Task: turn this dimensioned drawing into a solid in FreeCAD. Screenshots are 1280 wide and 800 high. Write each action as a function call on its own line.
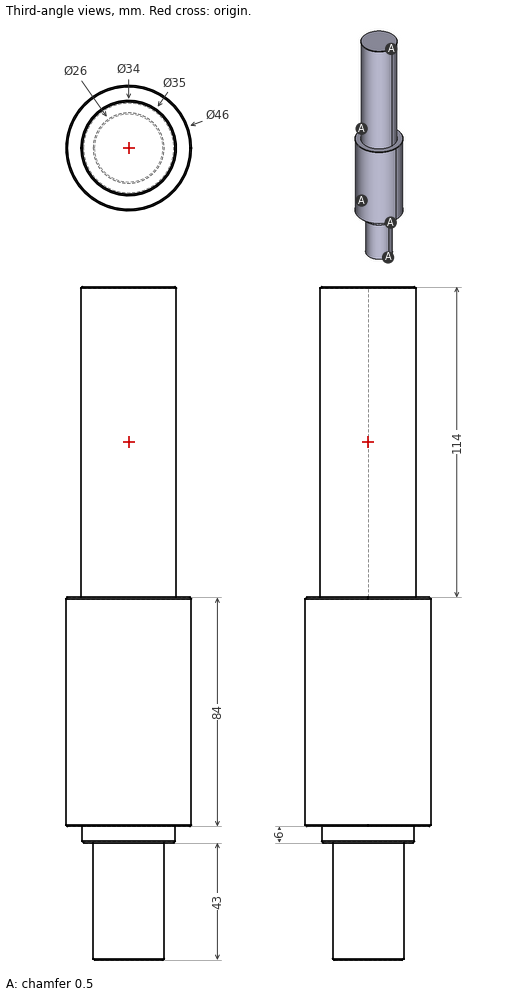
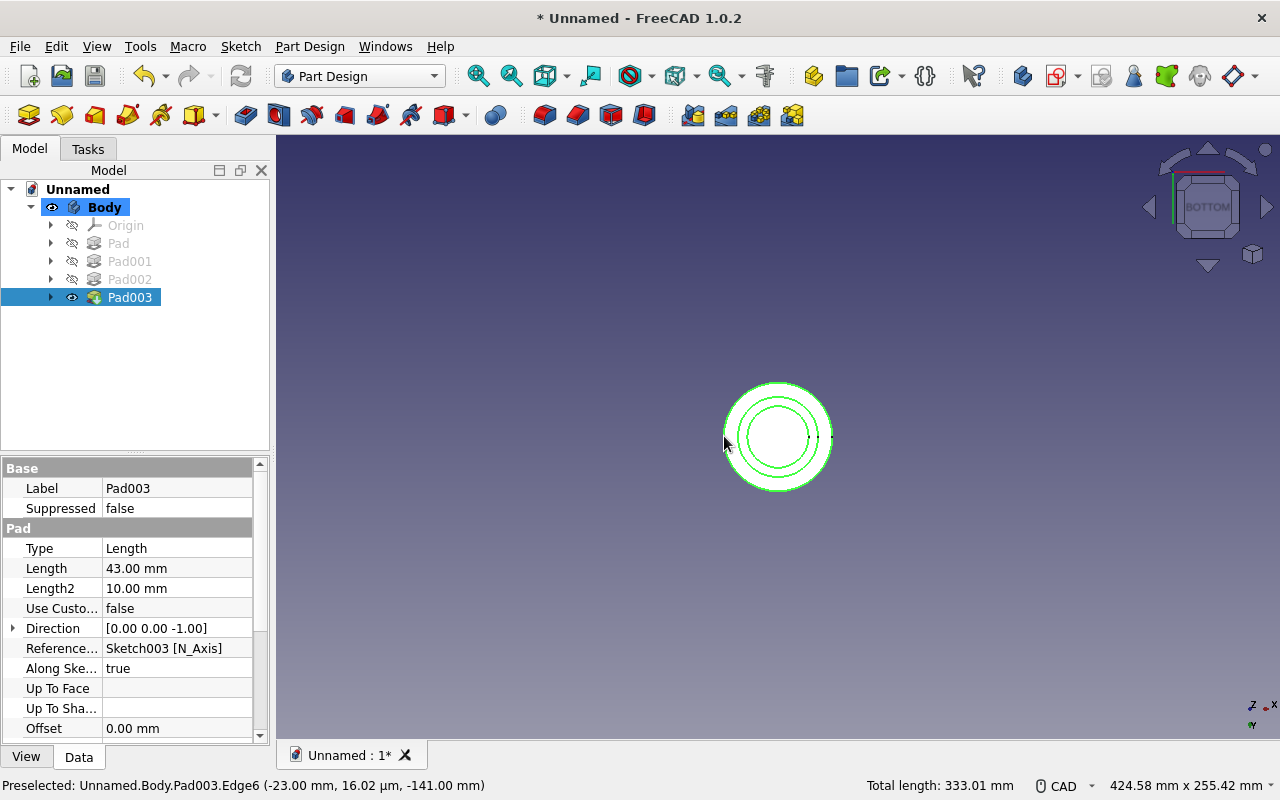
key(0)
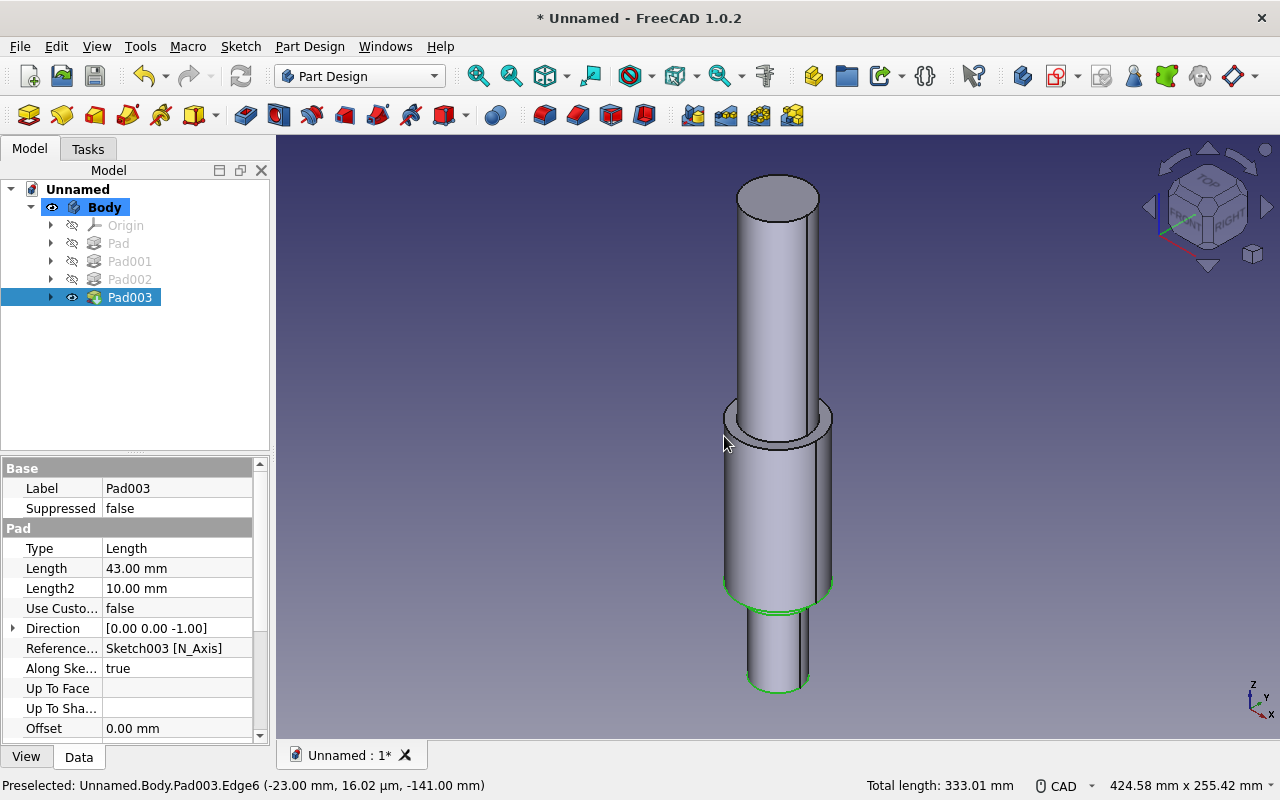
click(797, 176, ctrl)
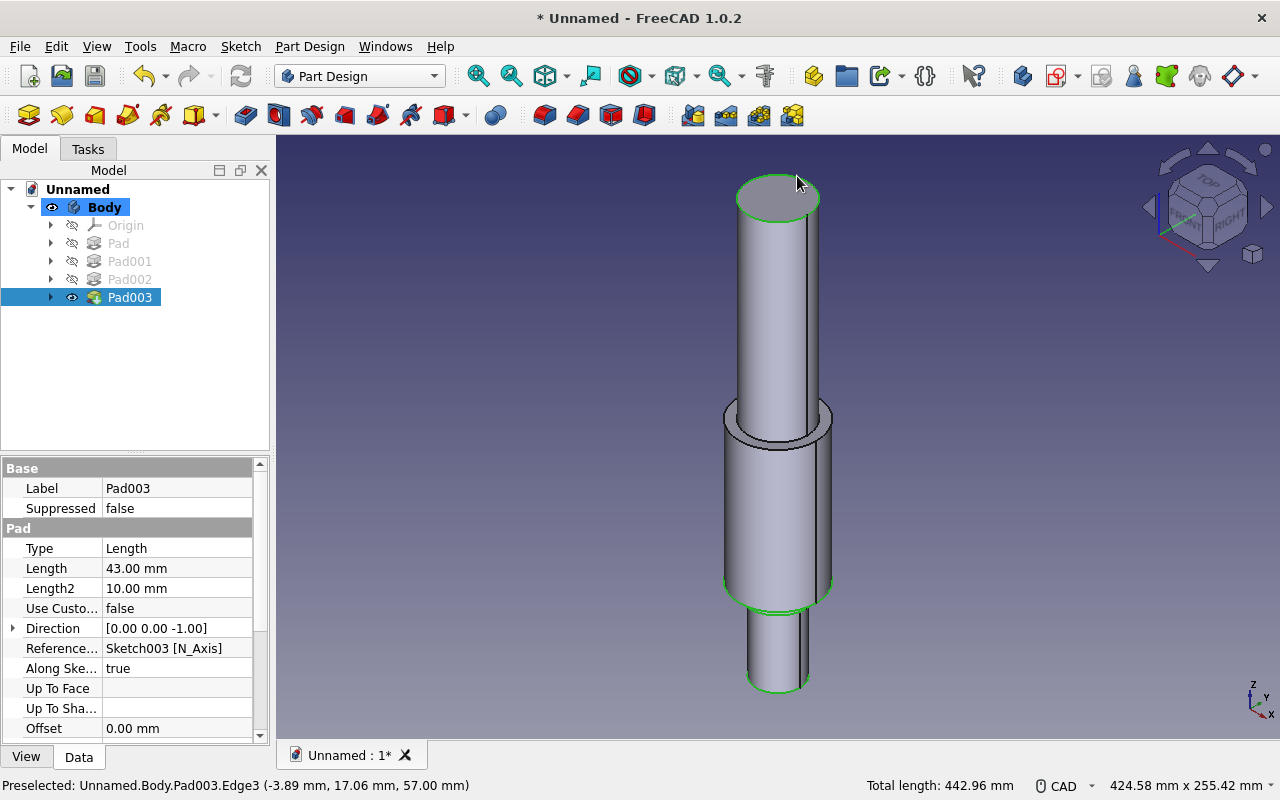
click(730, 432, ctrl)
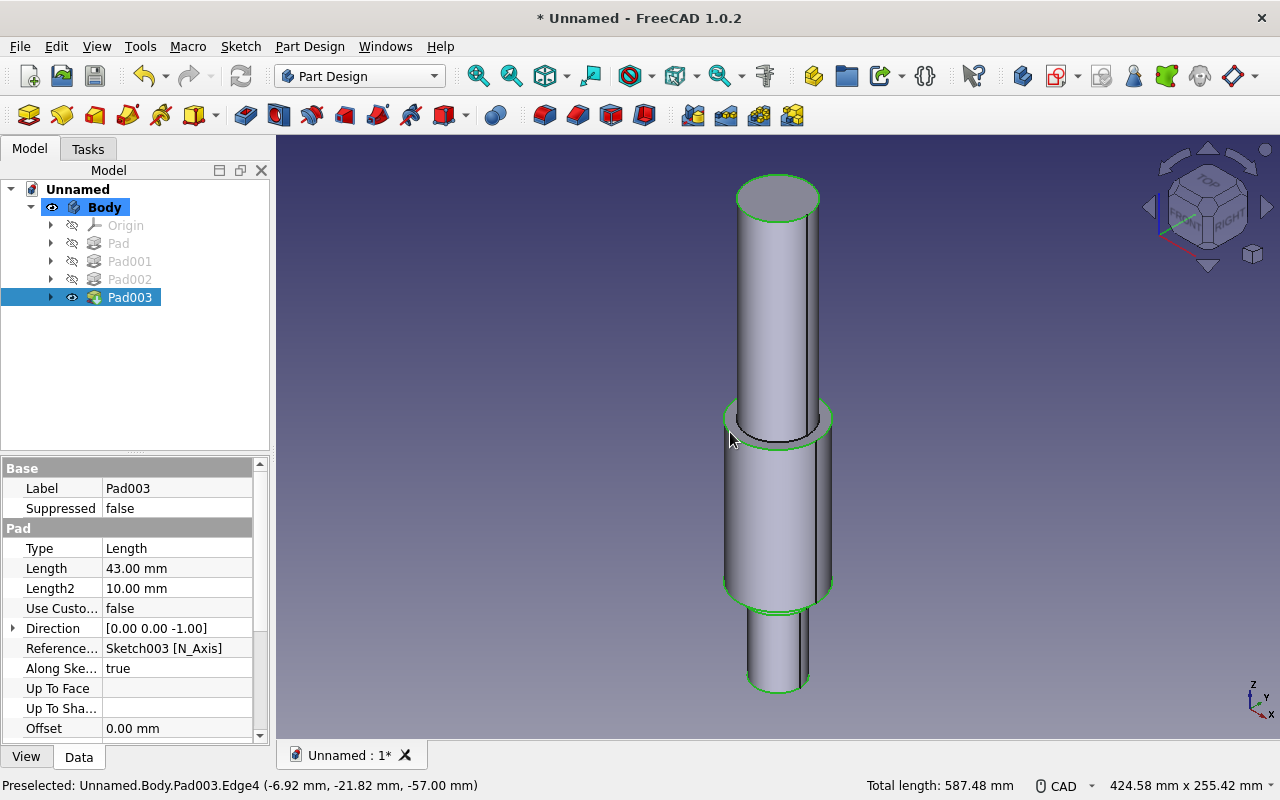
click(578, 116)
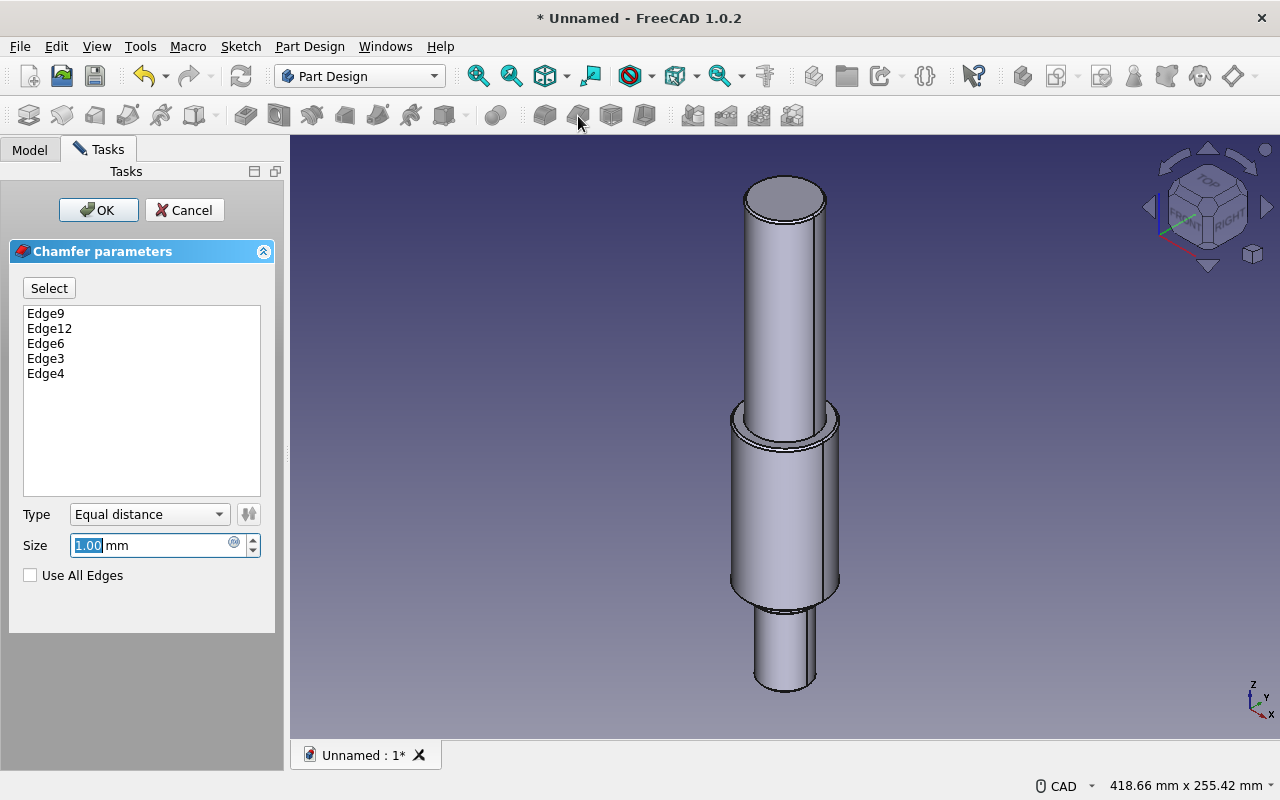
text(0.5)
key(Tab)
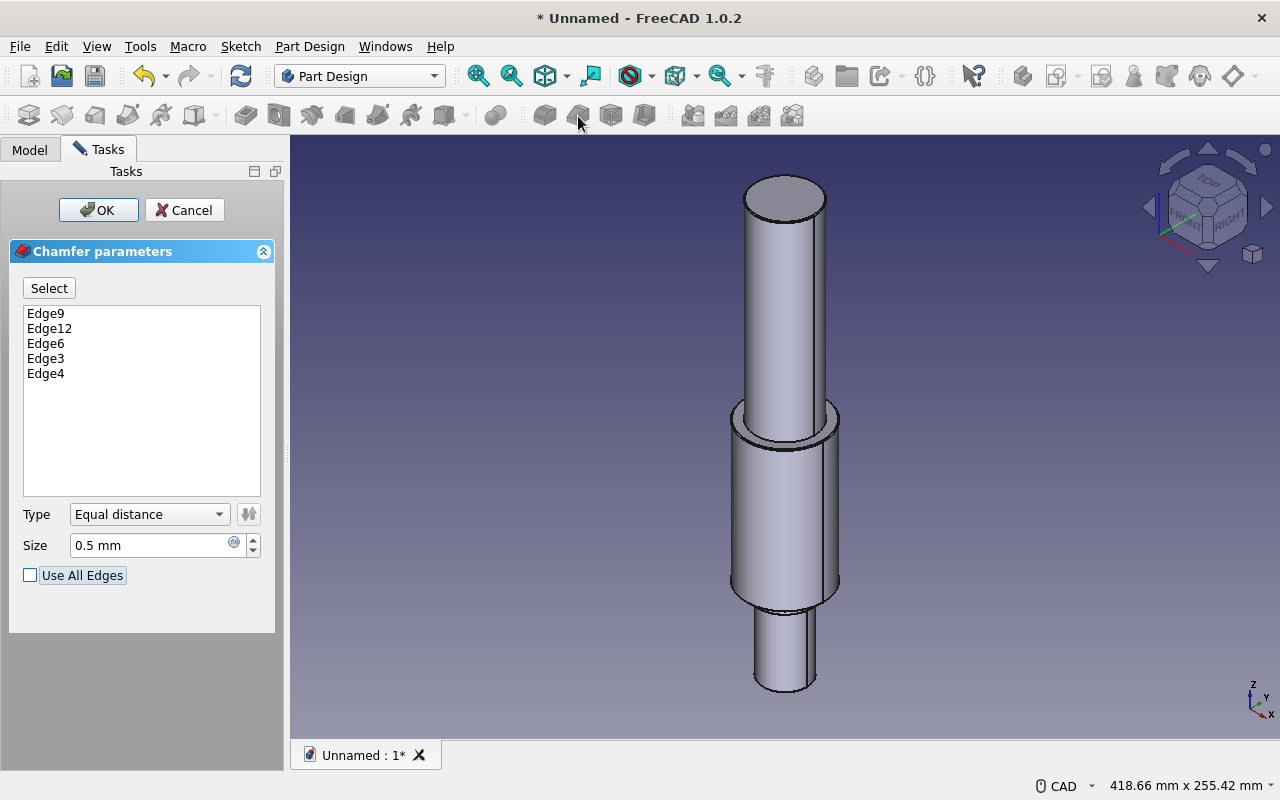
click(99, 210)